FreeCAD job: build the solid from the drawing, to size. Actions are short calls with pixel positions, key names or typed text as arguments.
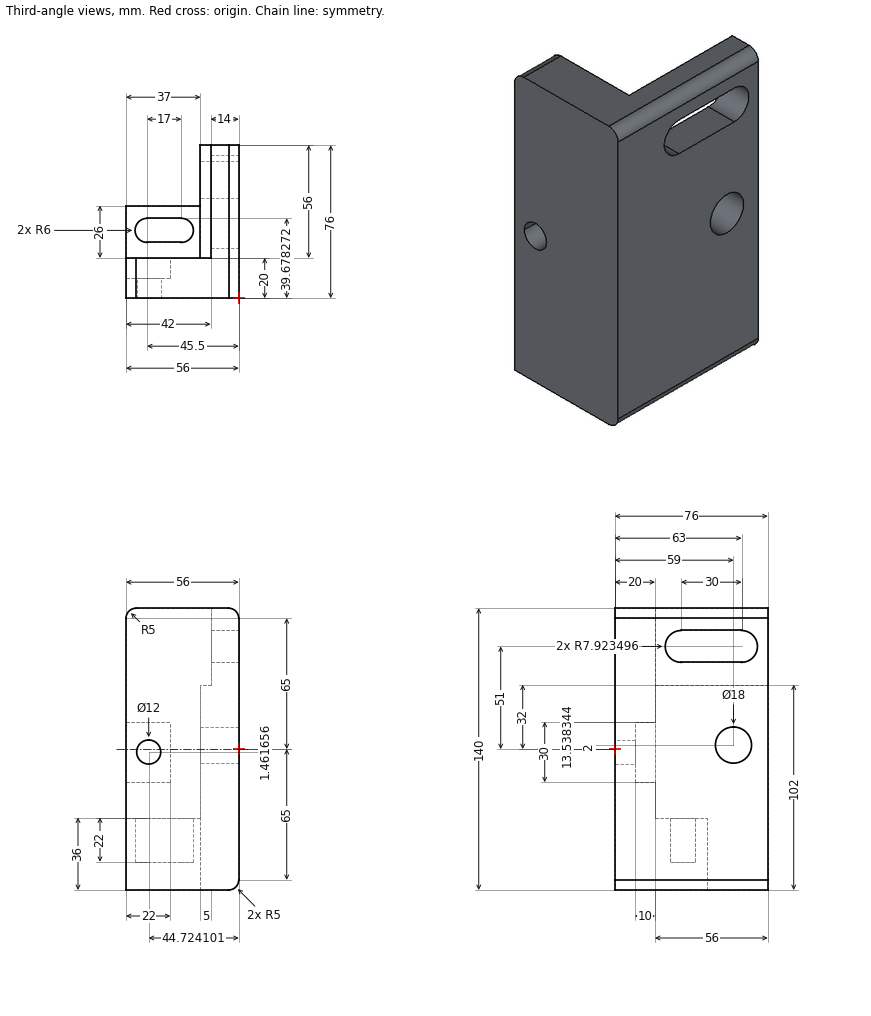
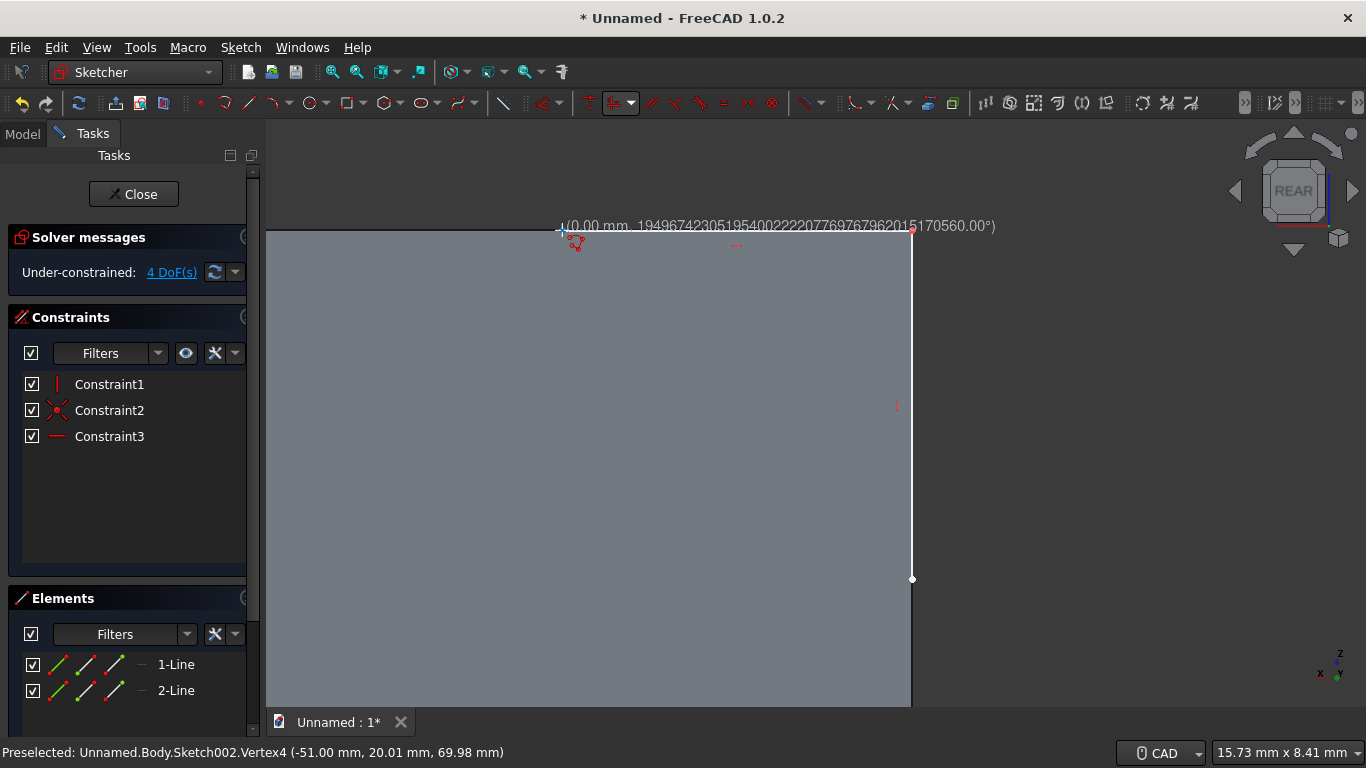
key(g)
key(3)
key(a)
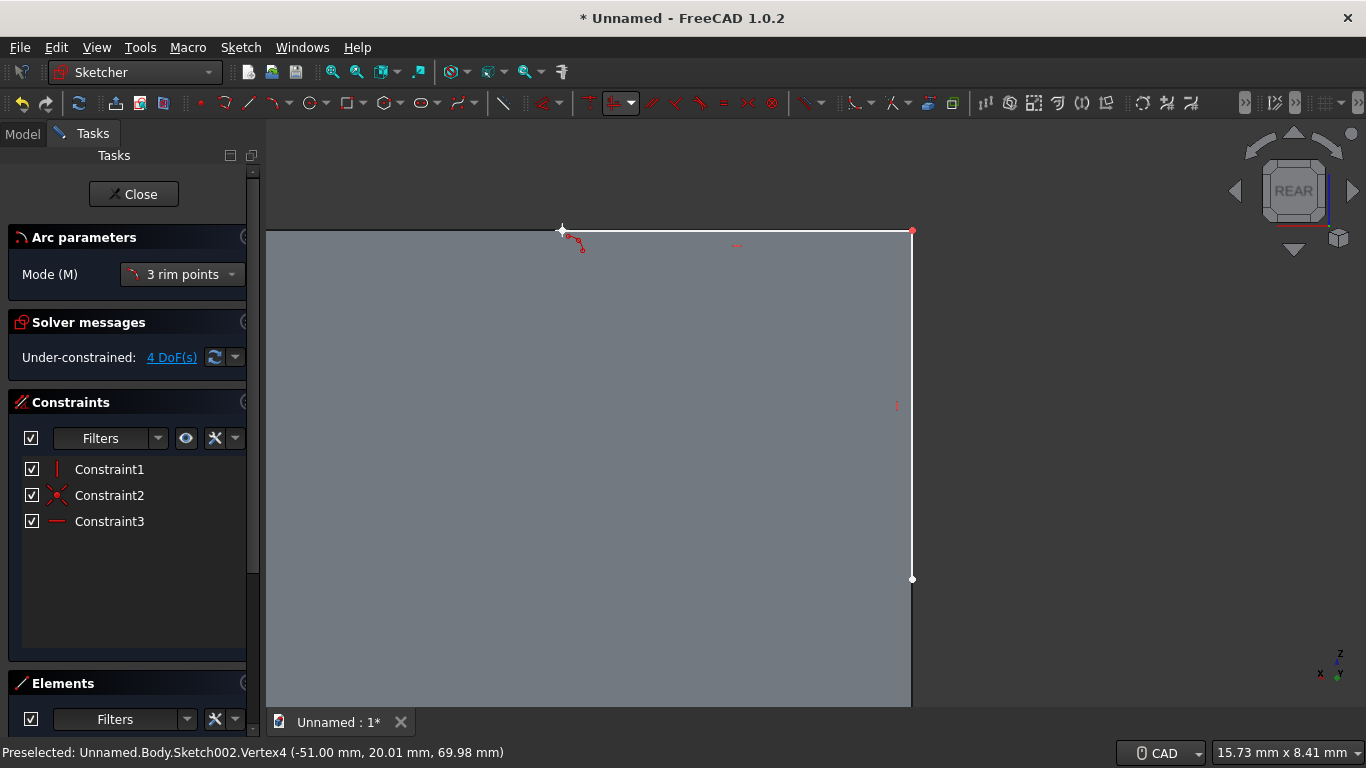
click(562, 231)
click(912, 580)
click(809, 332)
key(Escape)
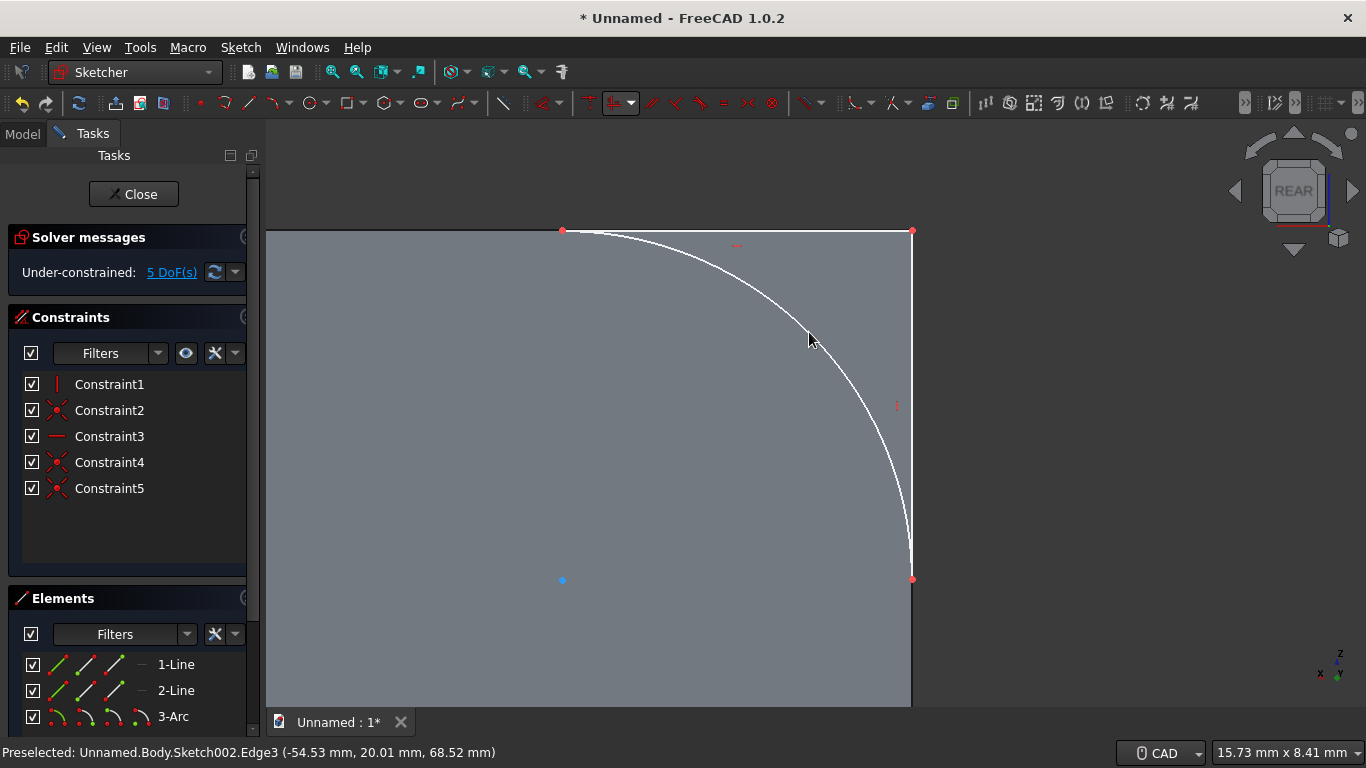
click(912, 475)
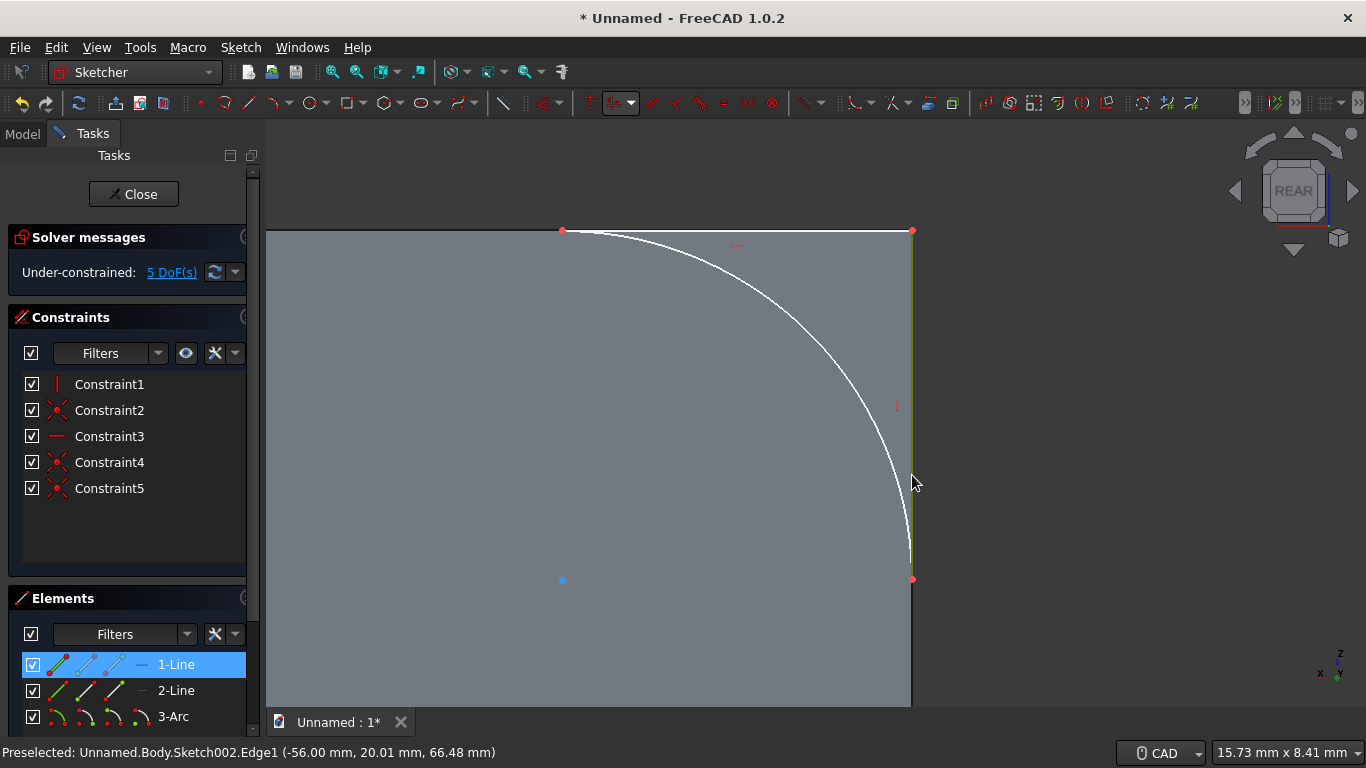
click(874, 421)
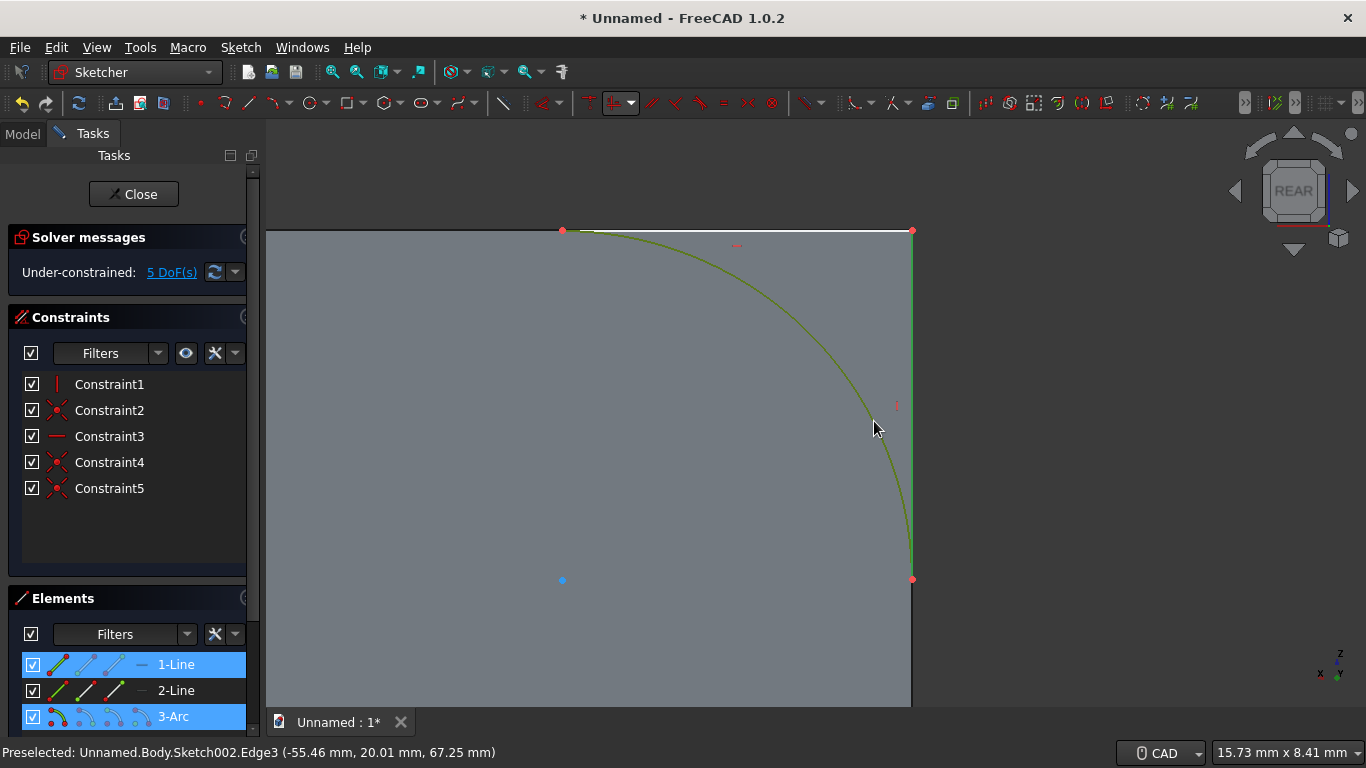
click(700, 104)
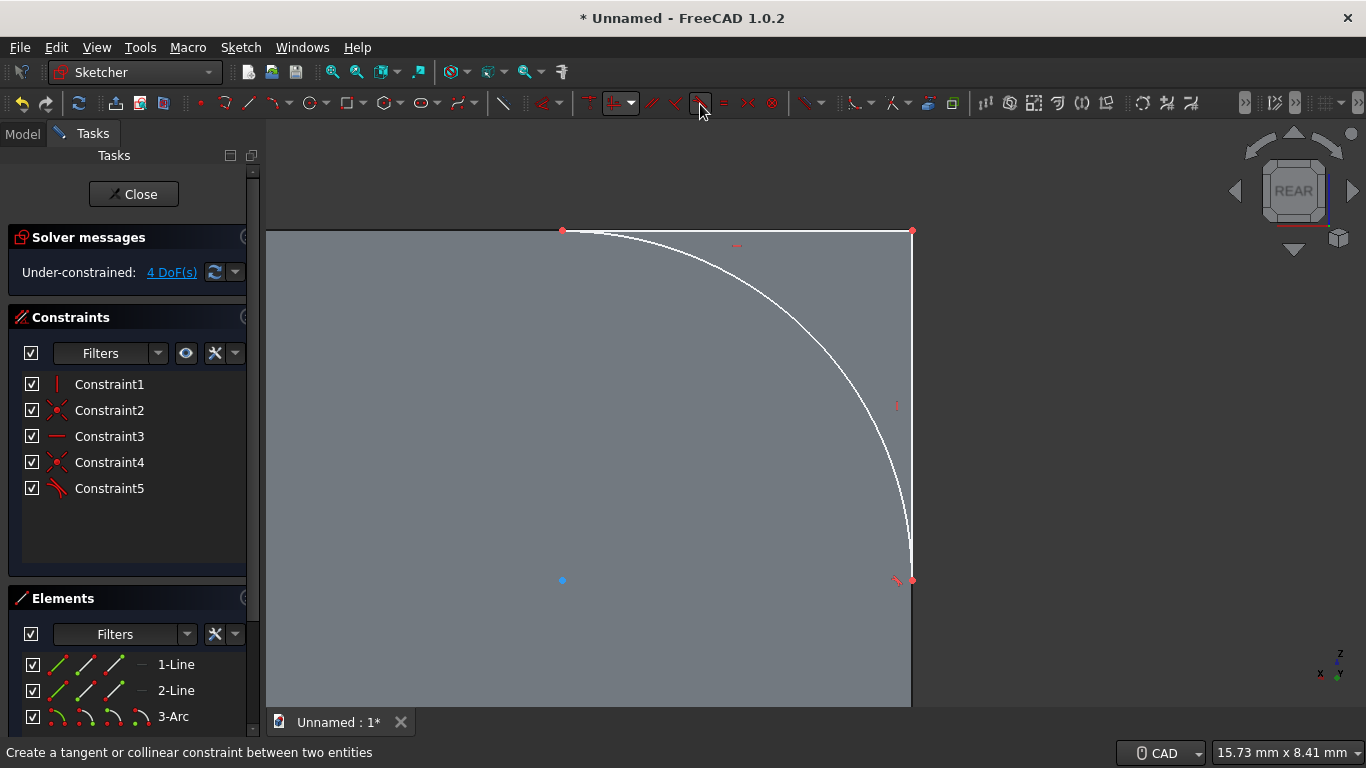
click(807, 231)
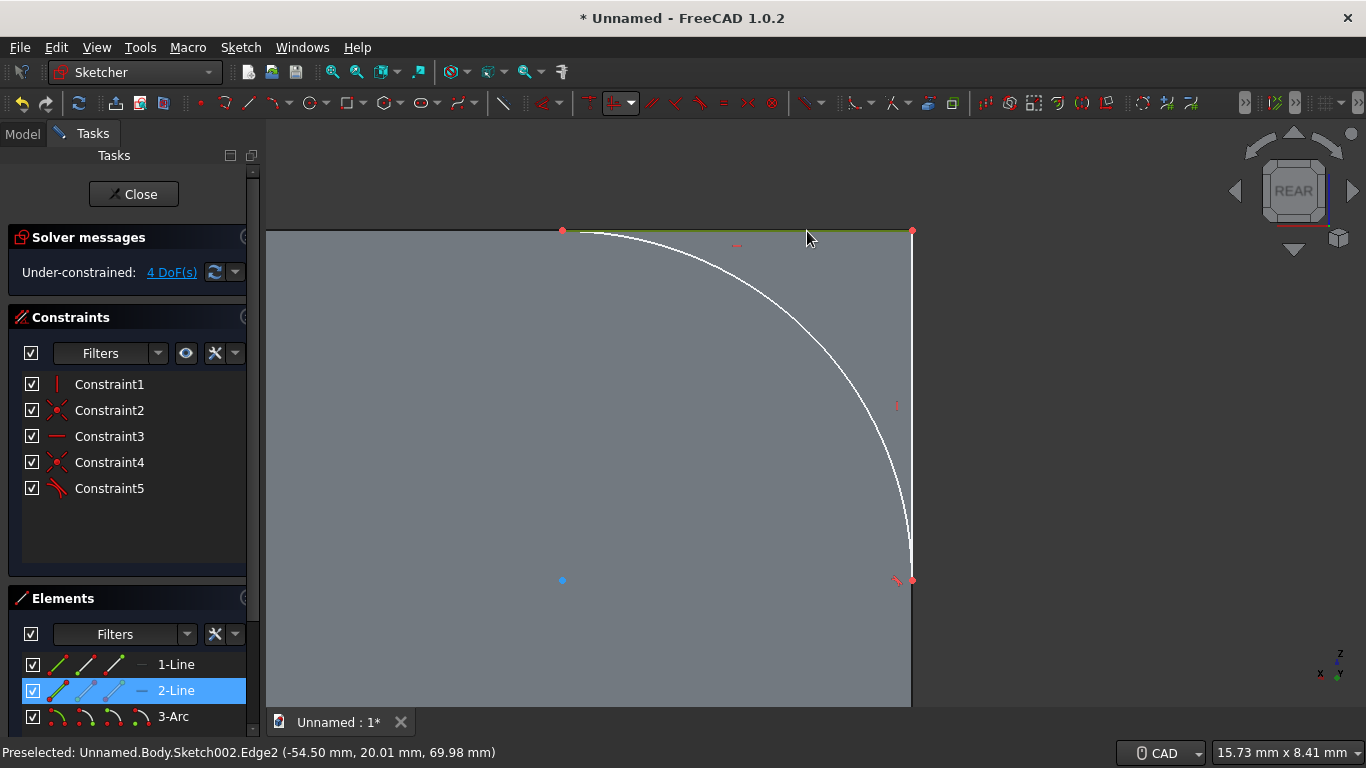
click(874, 422)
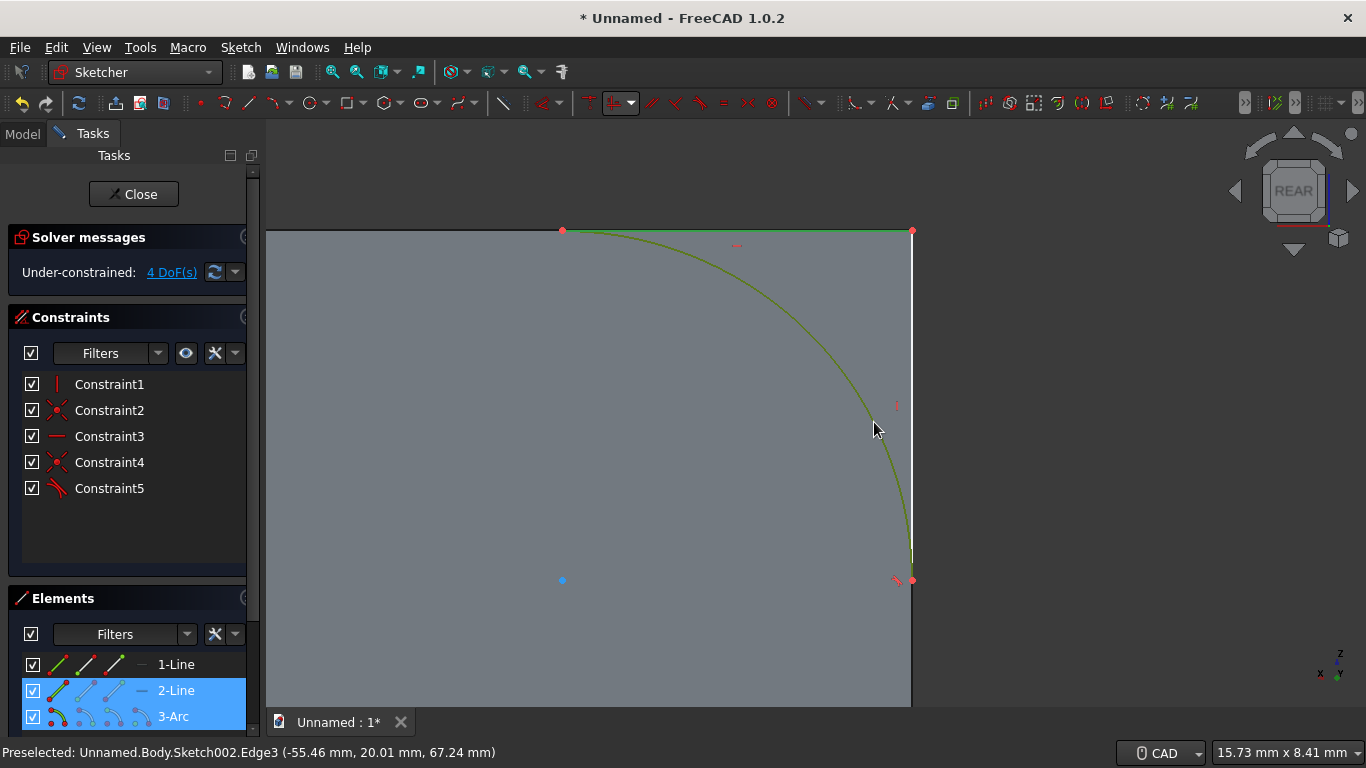
click(700, 104)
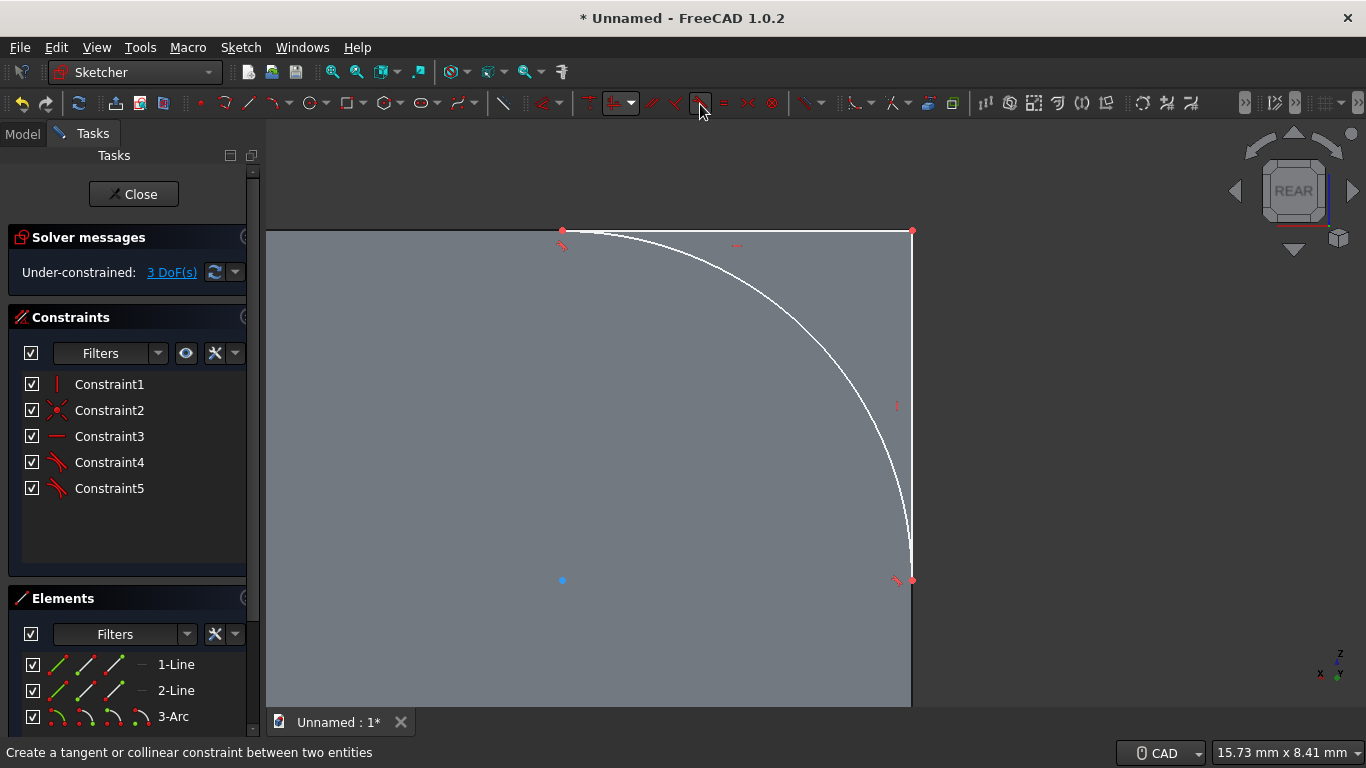
click(542, 104)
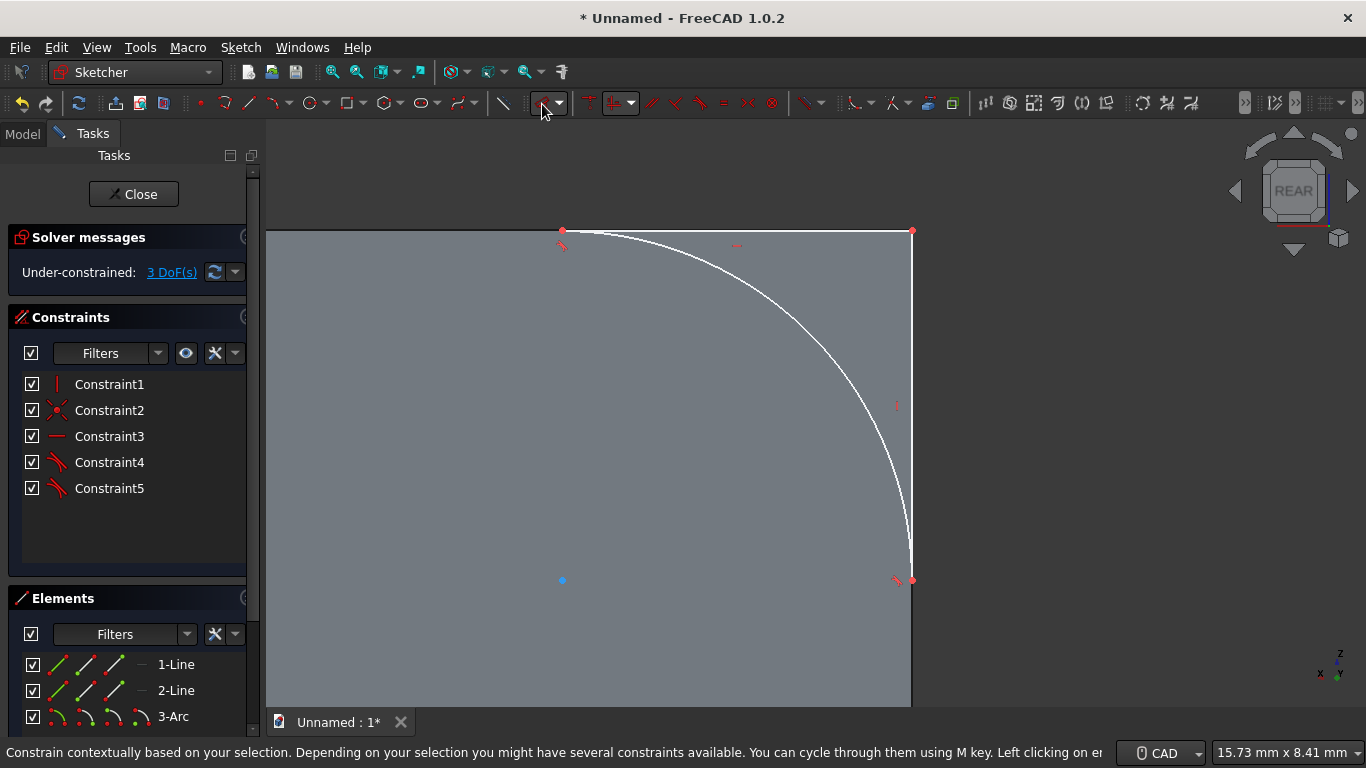
click(874, 422)
click(944, 592)